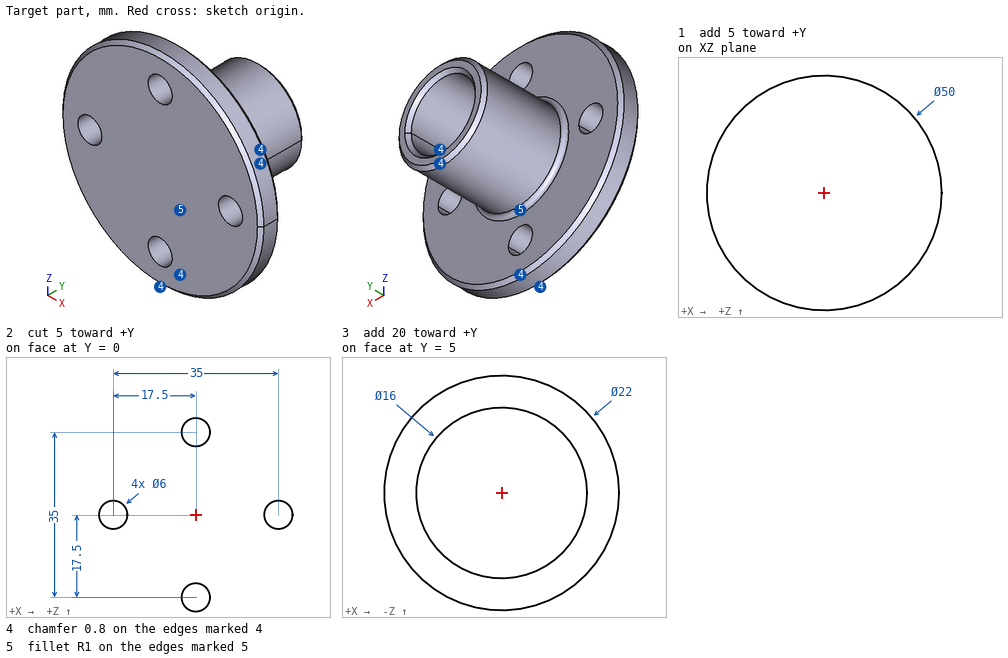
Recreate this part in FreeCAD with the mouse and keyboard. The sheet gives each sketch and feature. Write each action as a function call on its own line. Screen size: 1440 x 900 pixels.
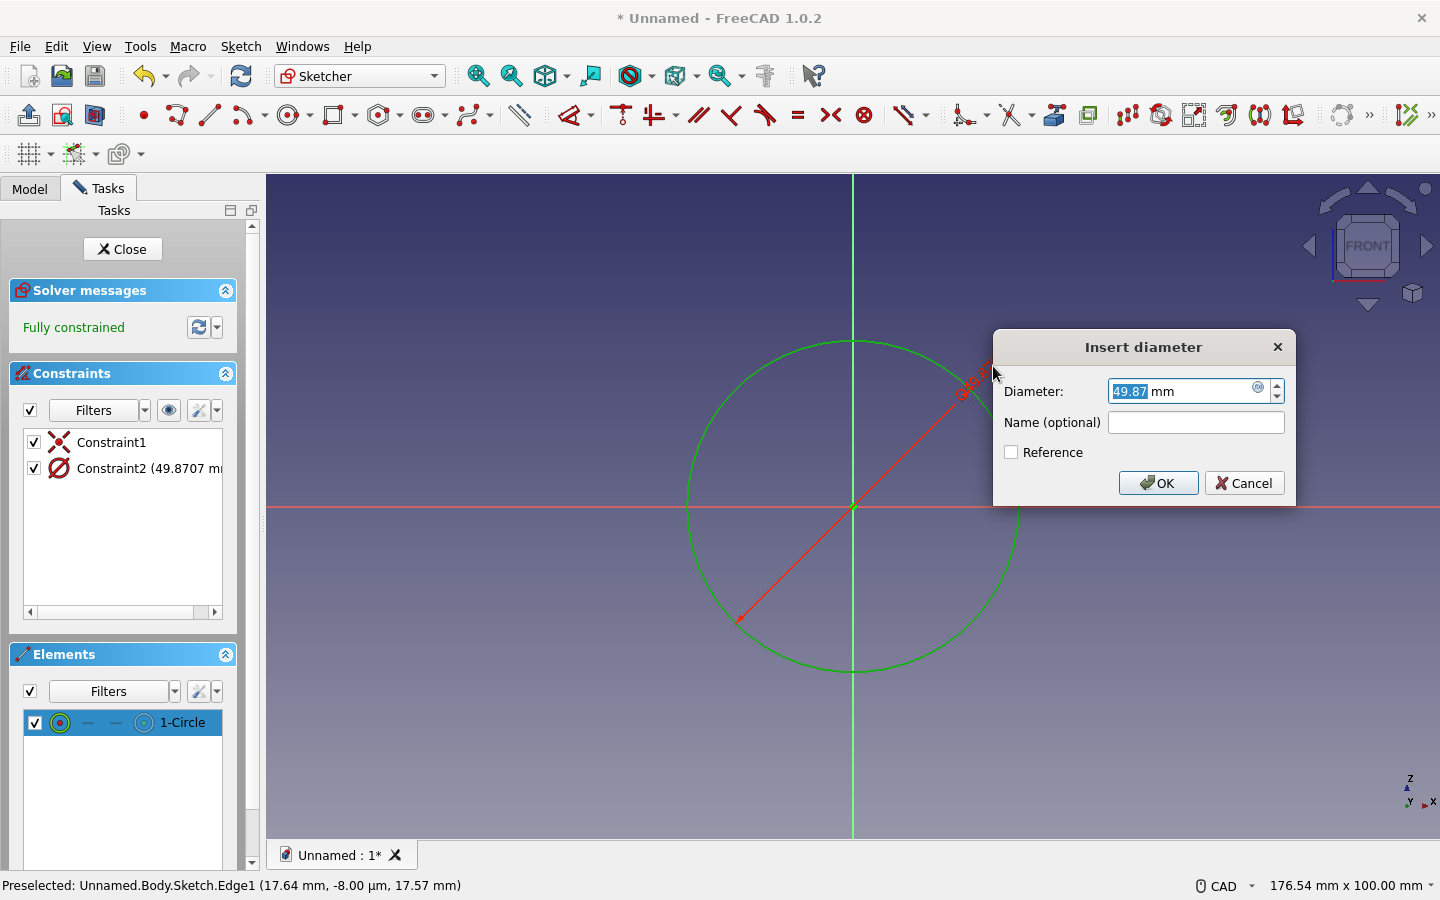
text(50)
key(Return)
key(Escape)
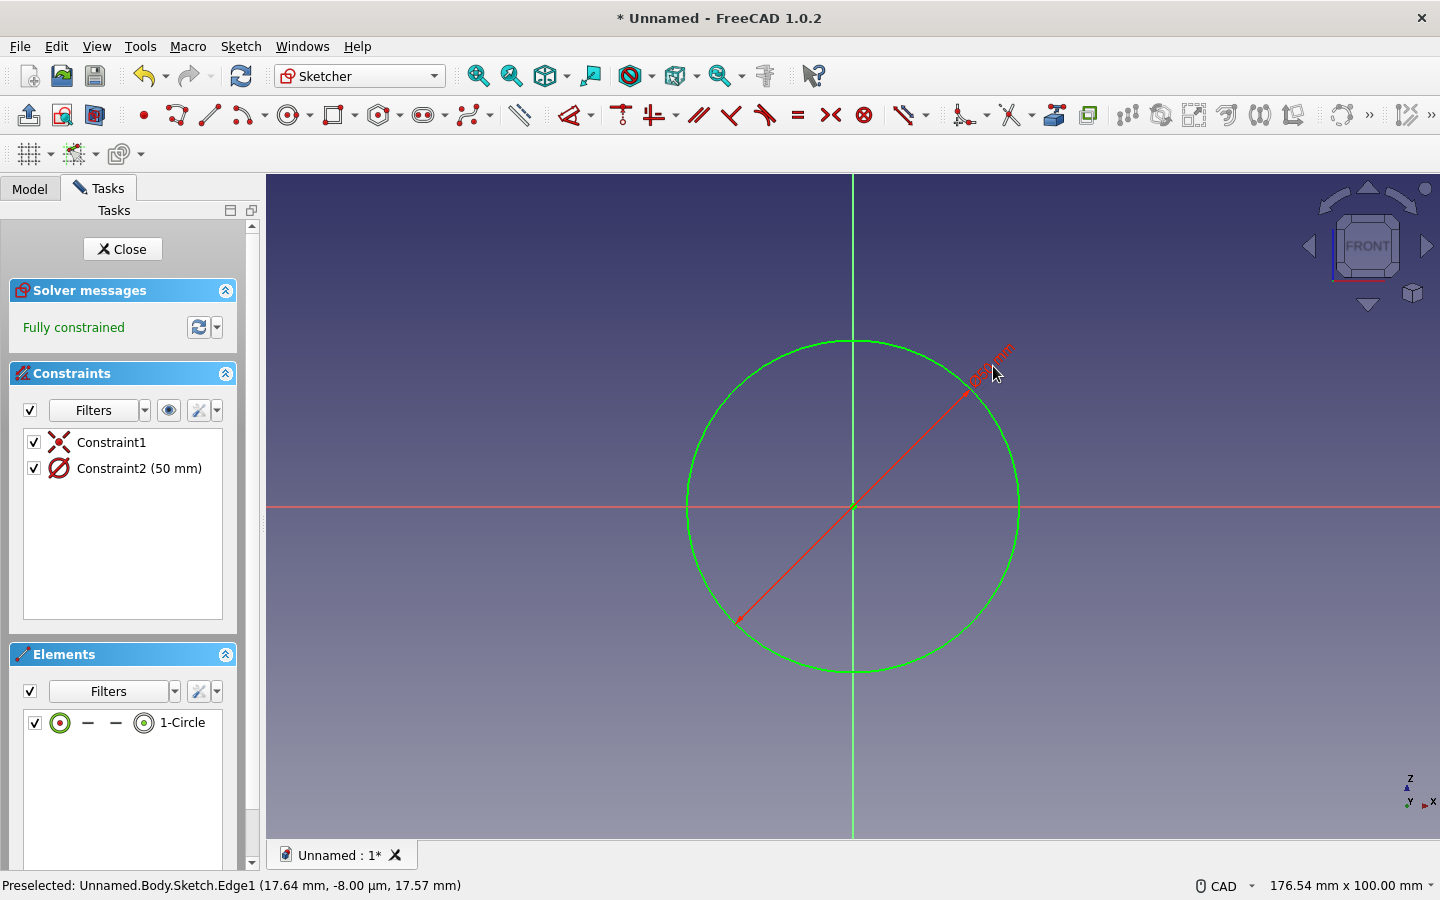
click(123, 249)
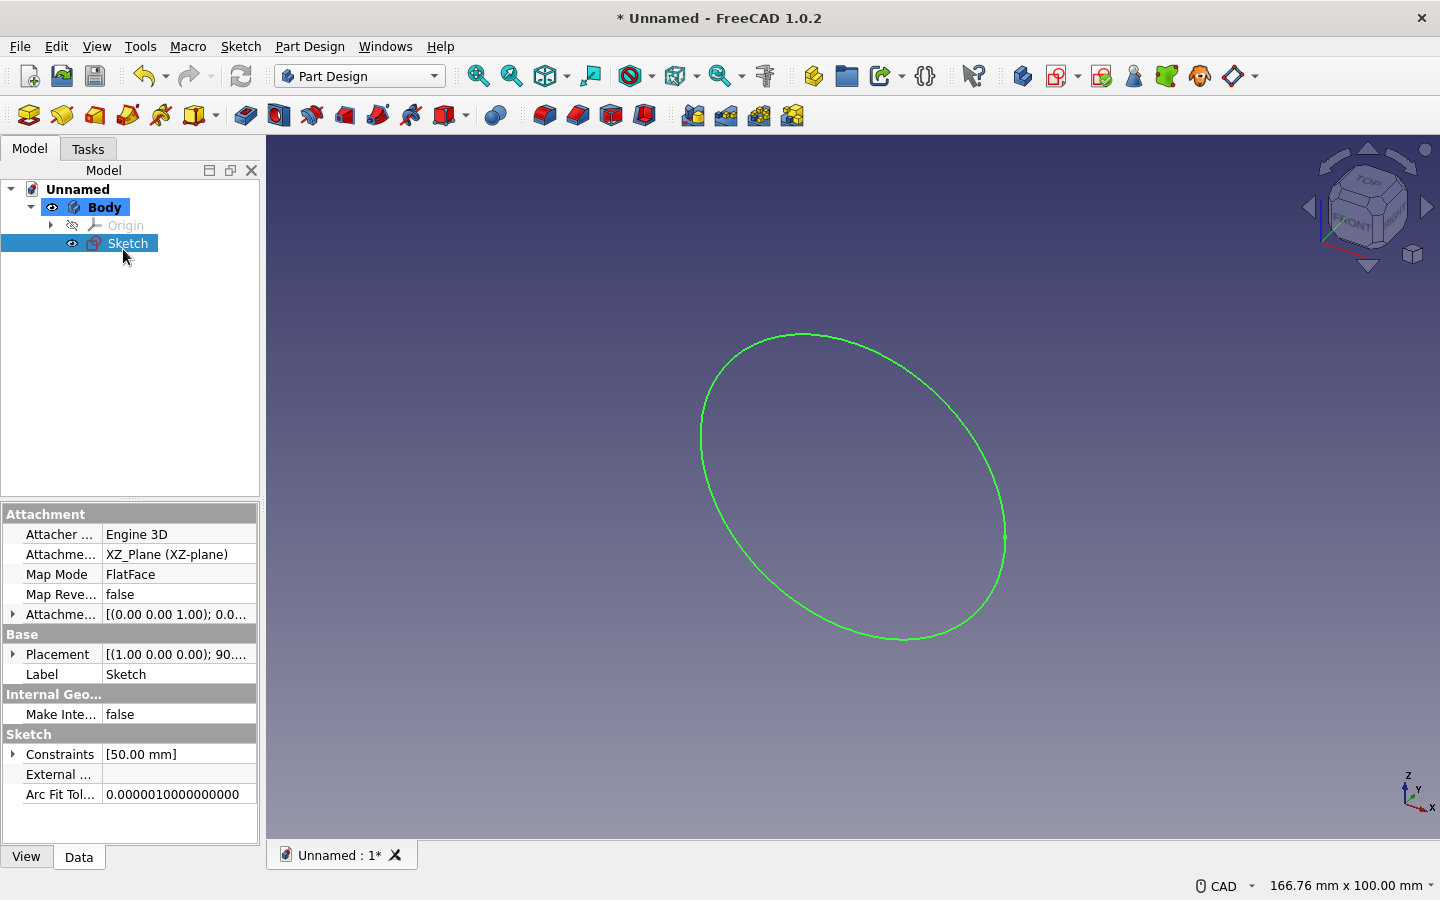
click(29, 116)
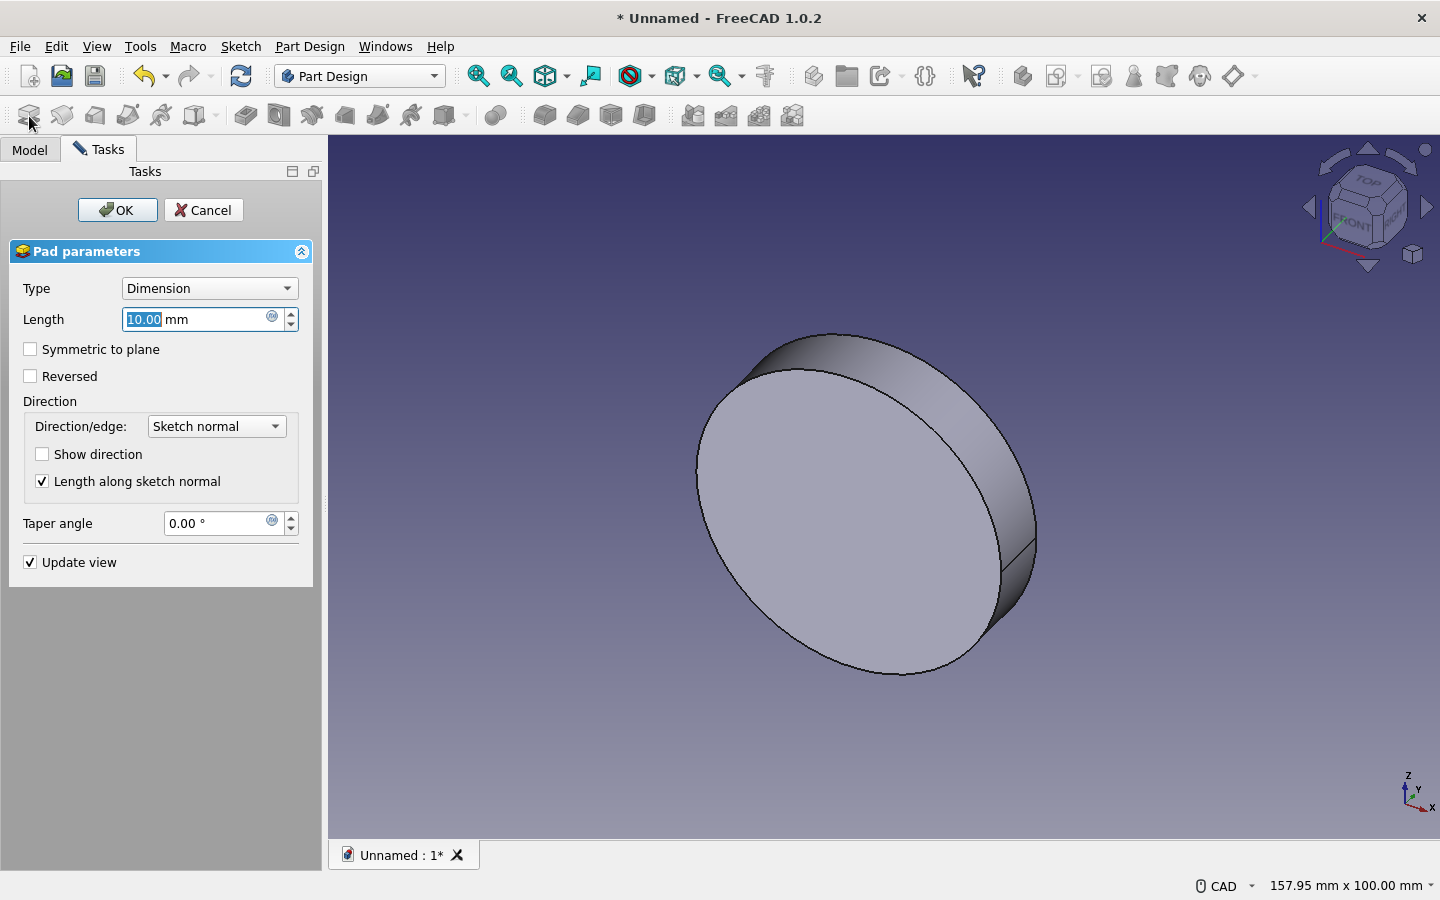
text(5)
key(Tab)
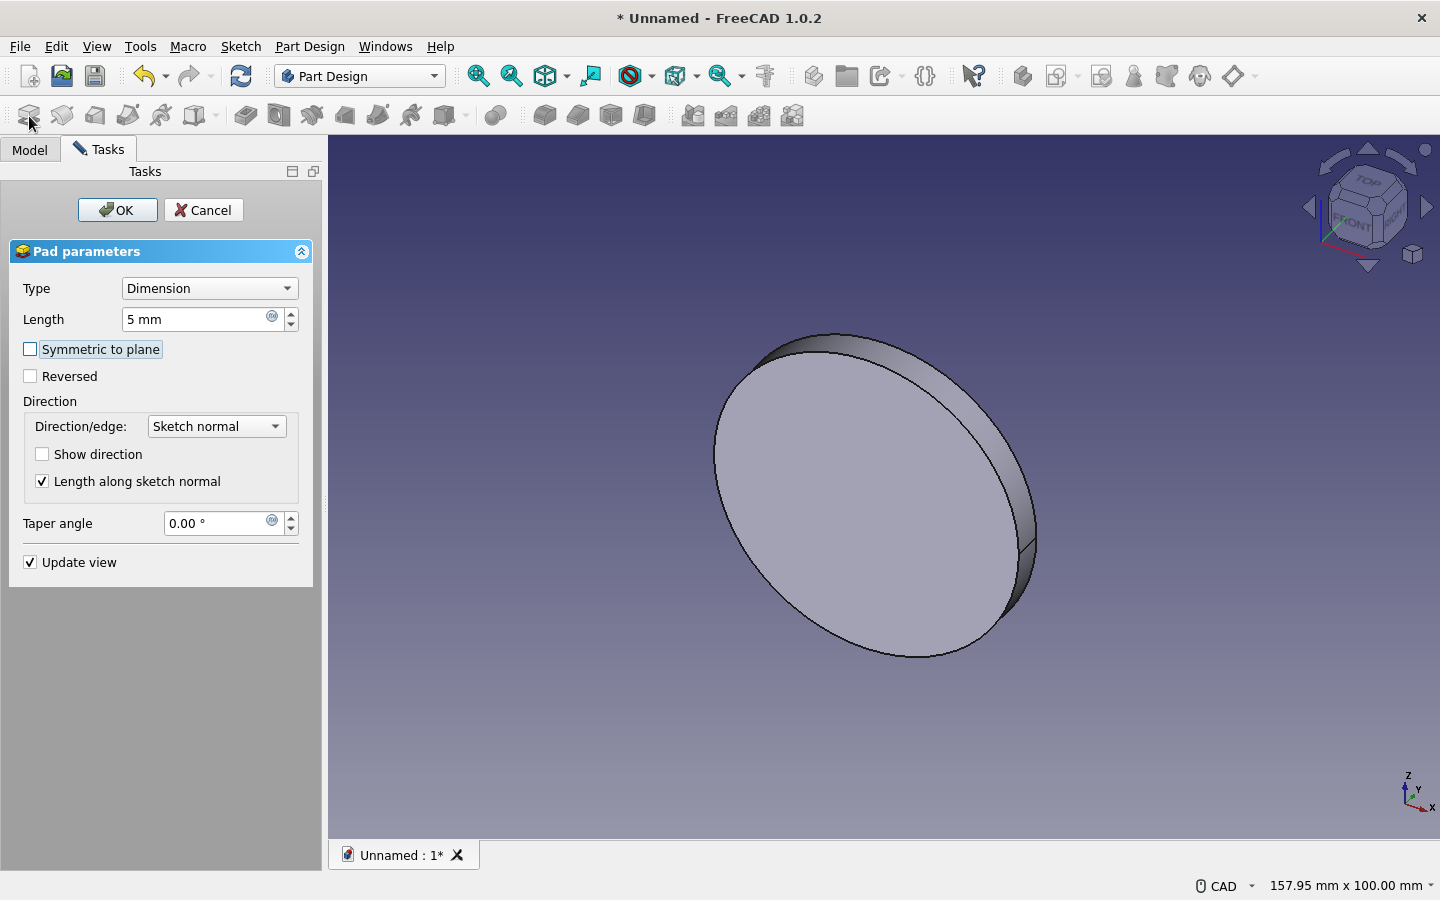
click(31, 376)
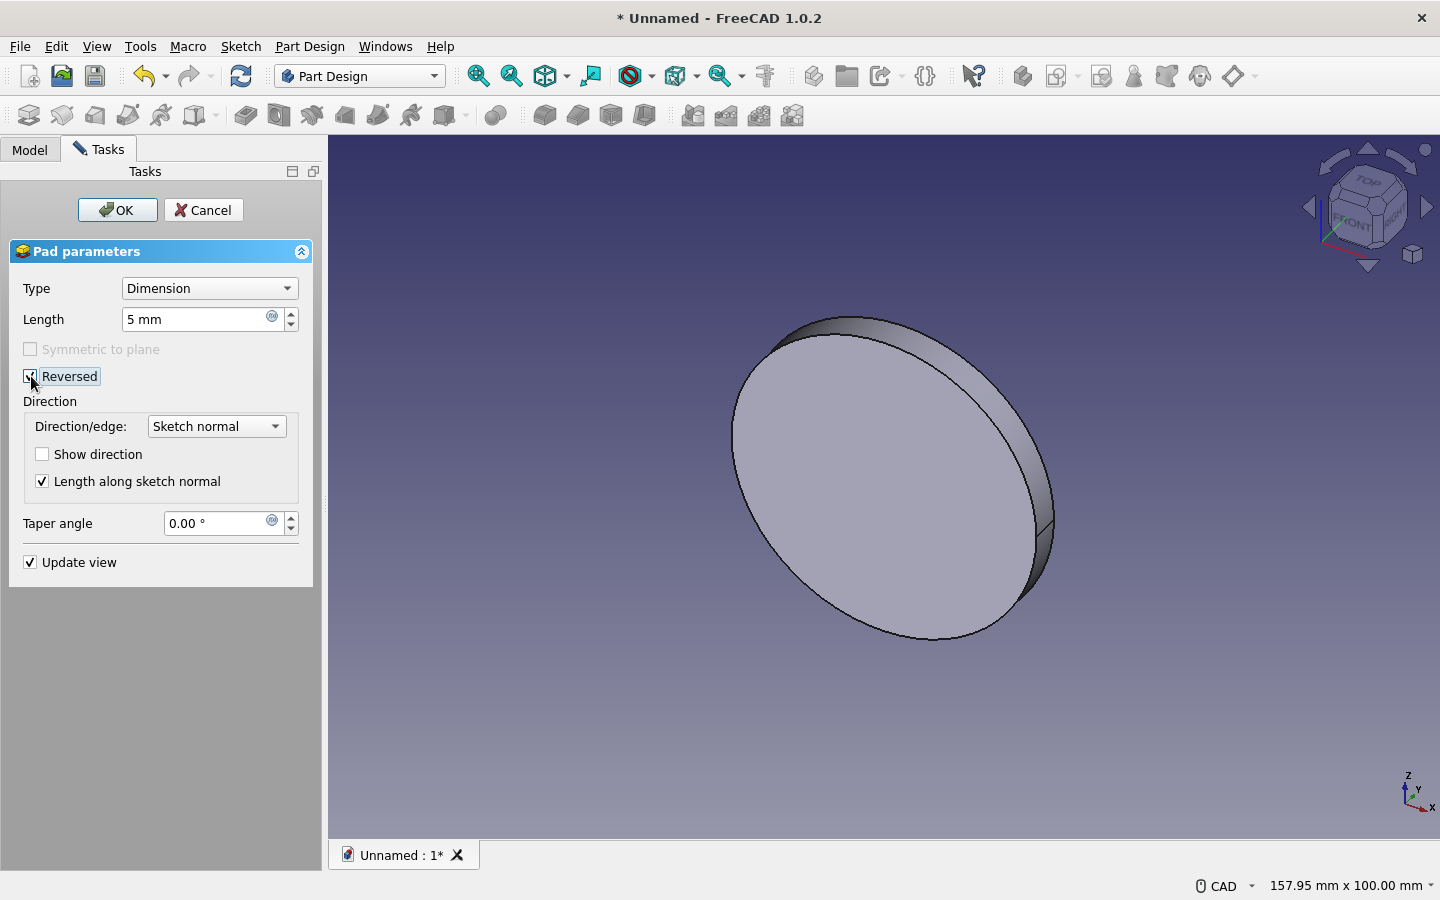
click(118, 210)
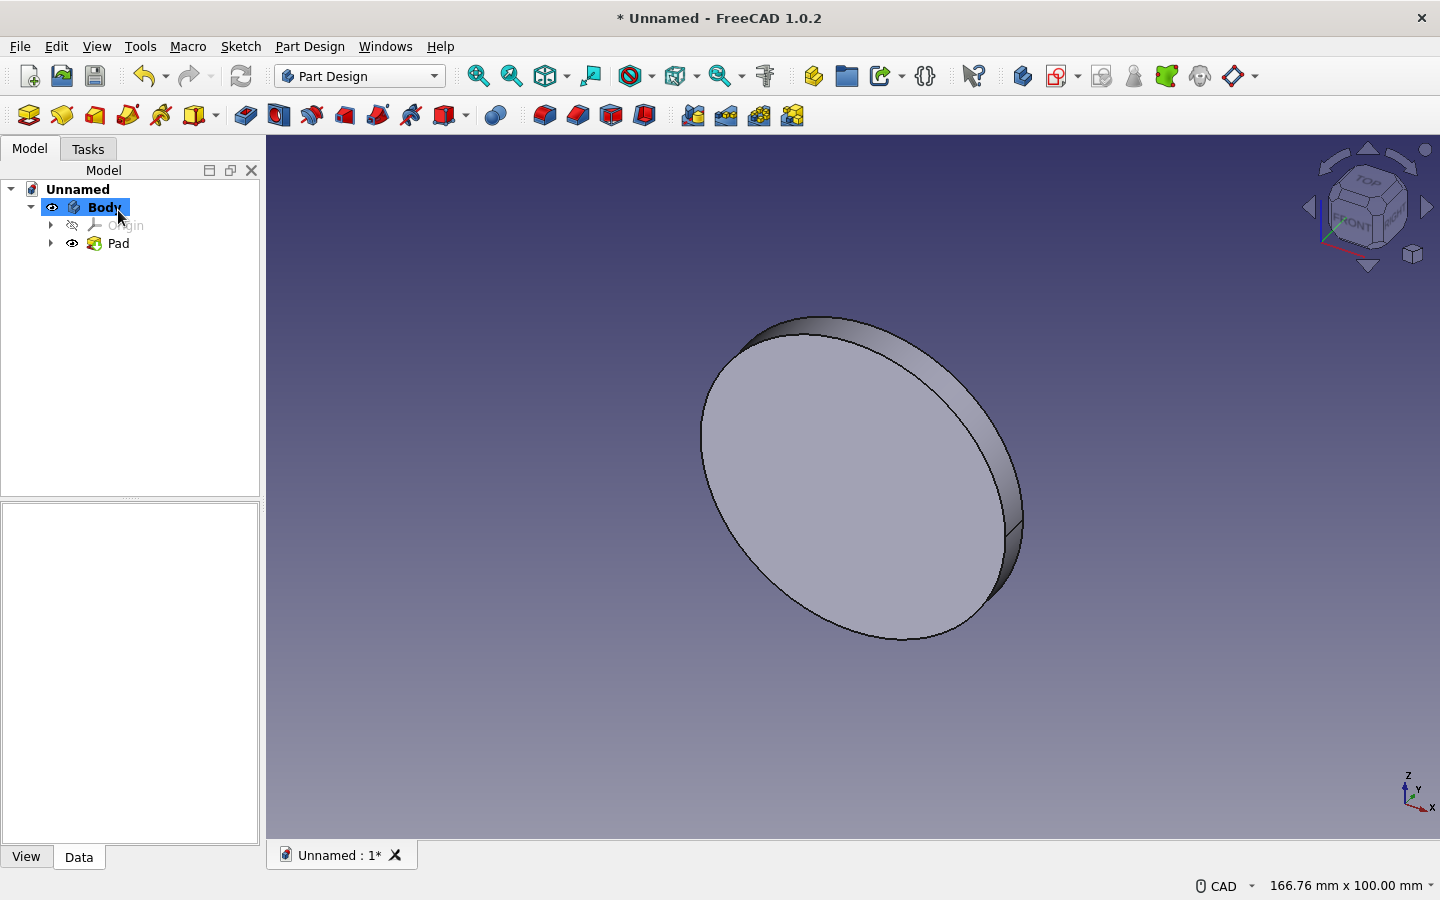
click(853, 486)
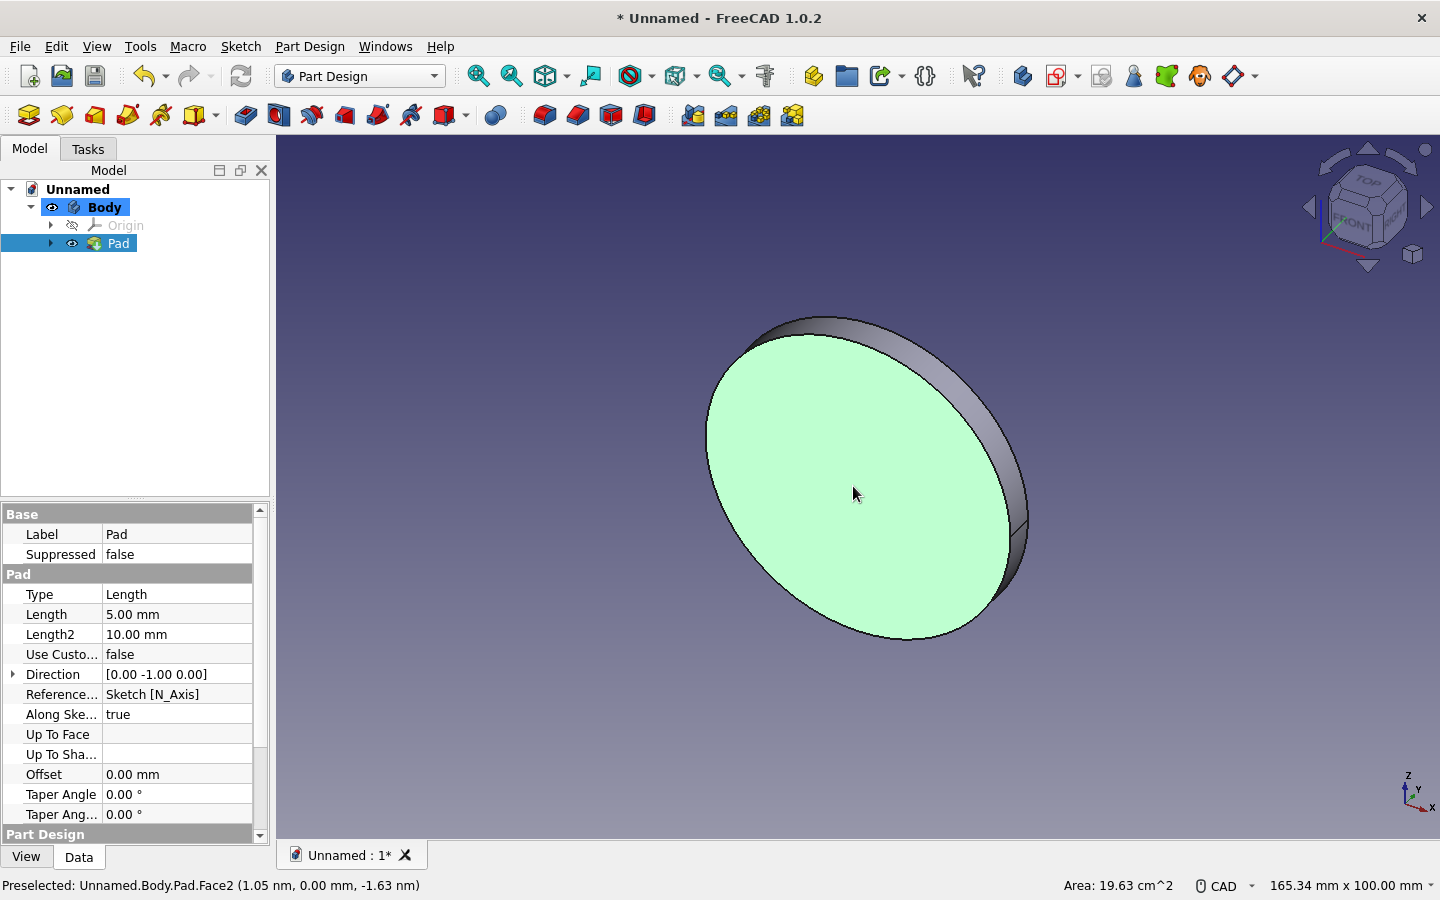
click(1056, 76)